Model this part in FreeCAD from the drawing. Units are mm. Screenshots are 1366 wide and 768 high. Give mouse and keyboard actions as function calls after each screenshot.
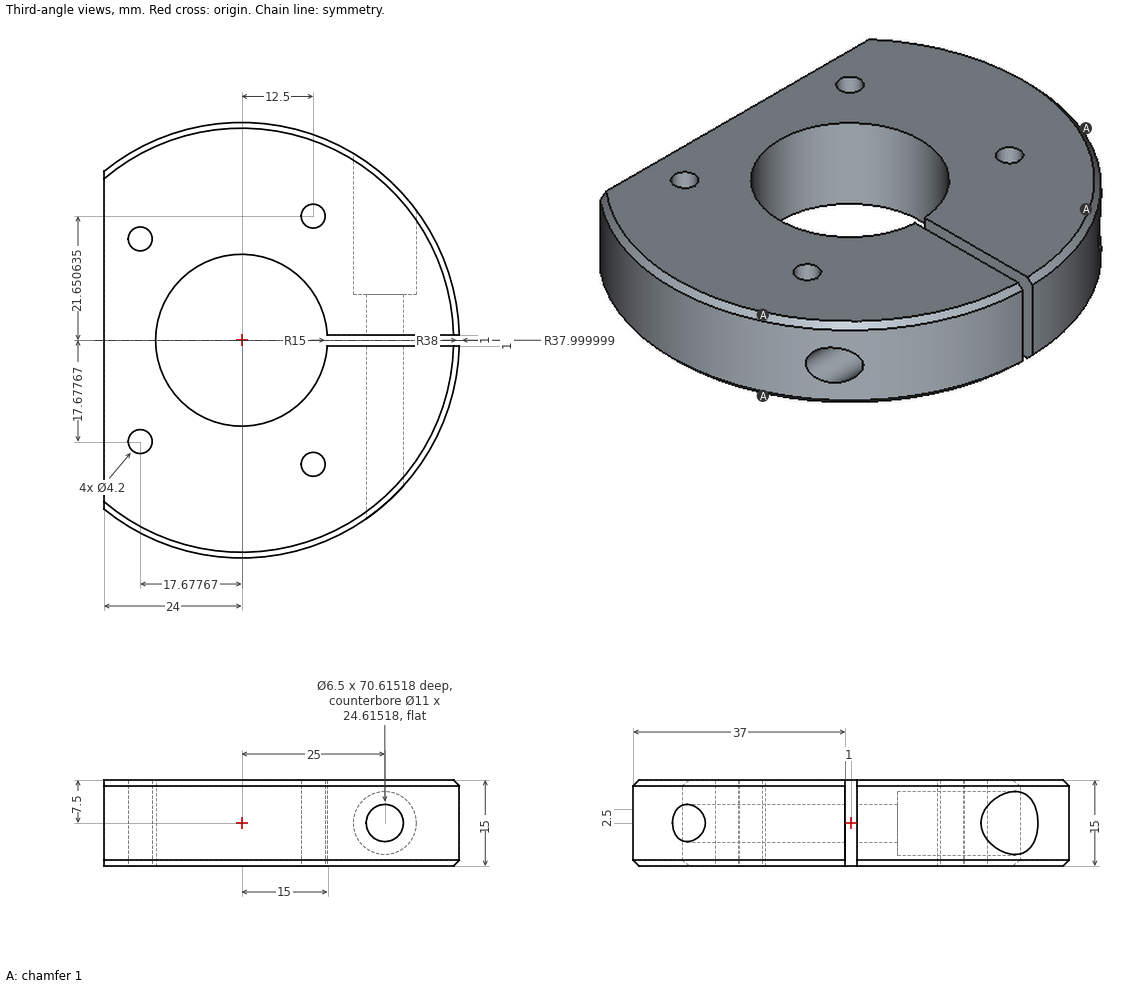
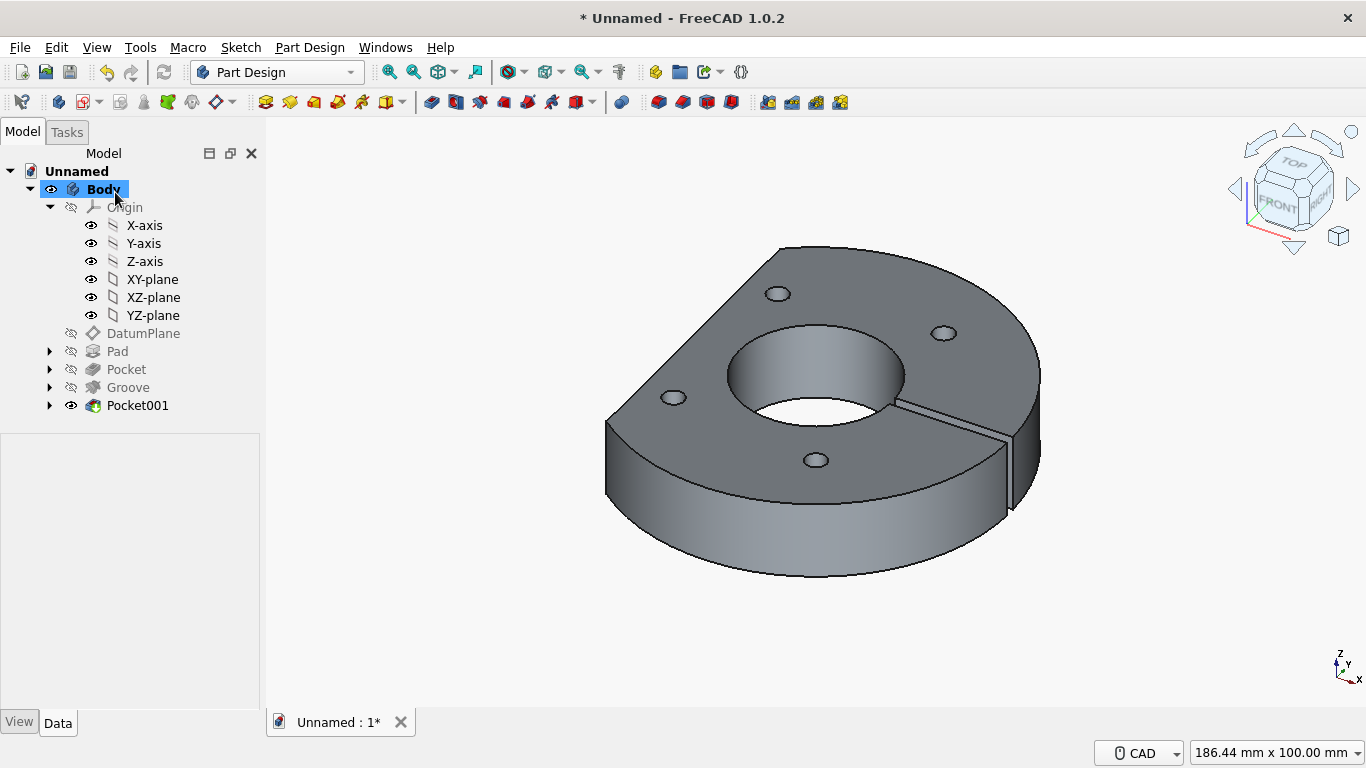
click(136, 315)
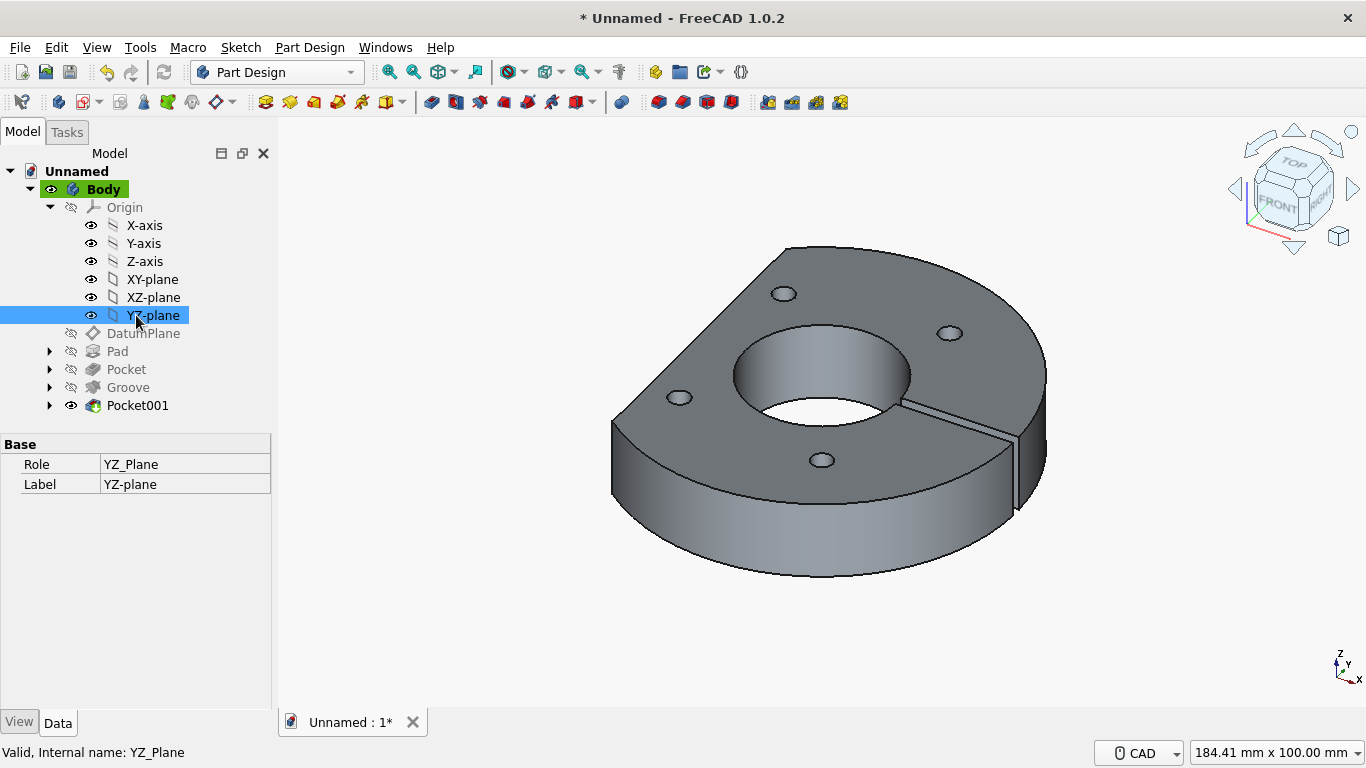
click(216, 102)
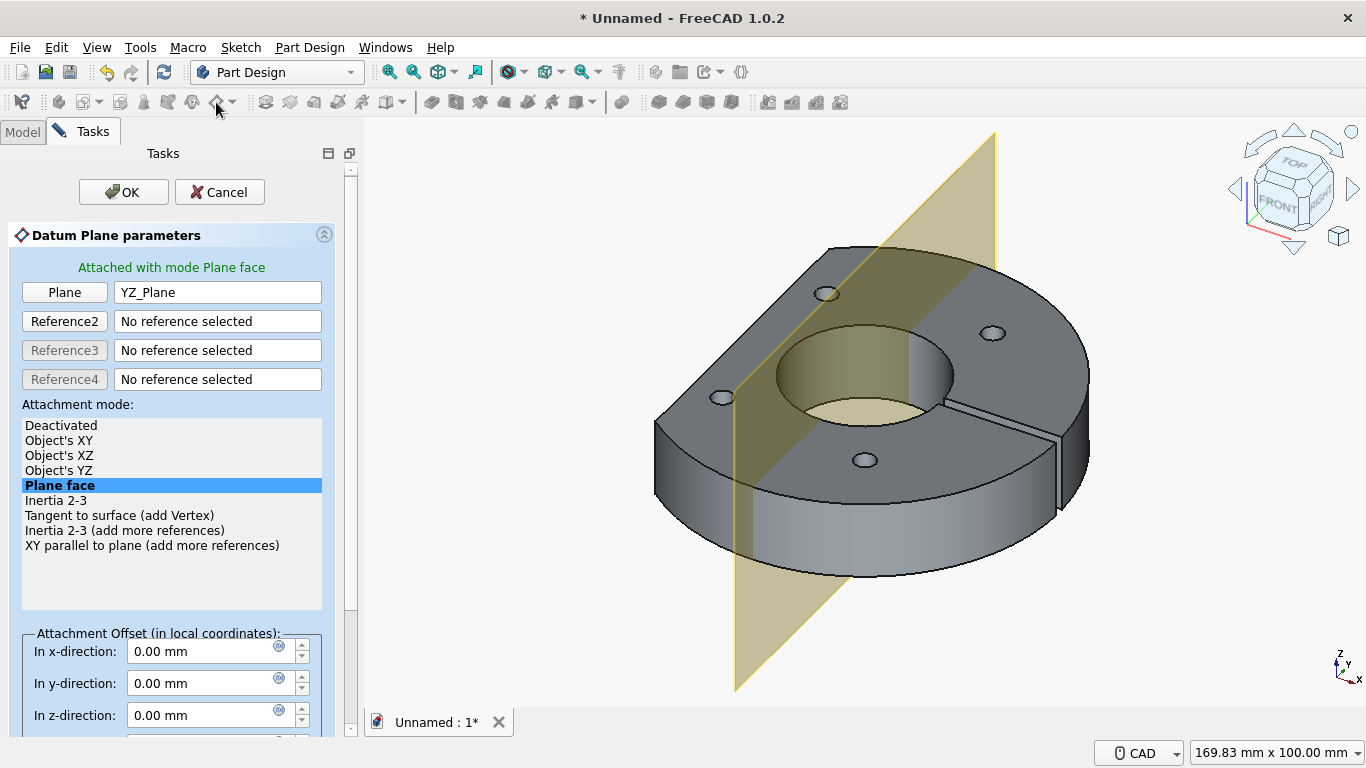
triple_click(210, 715)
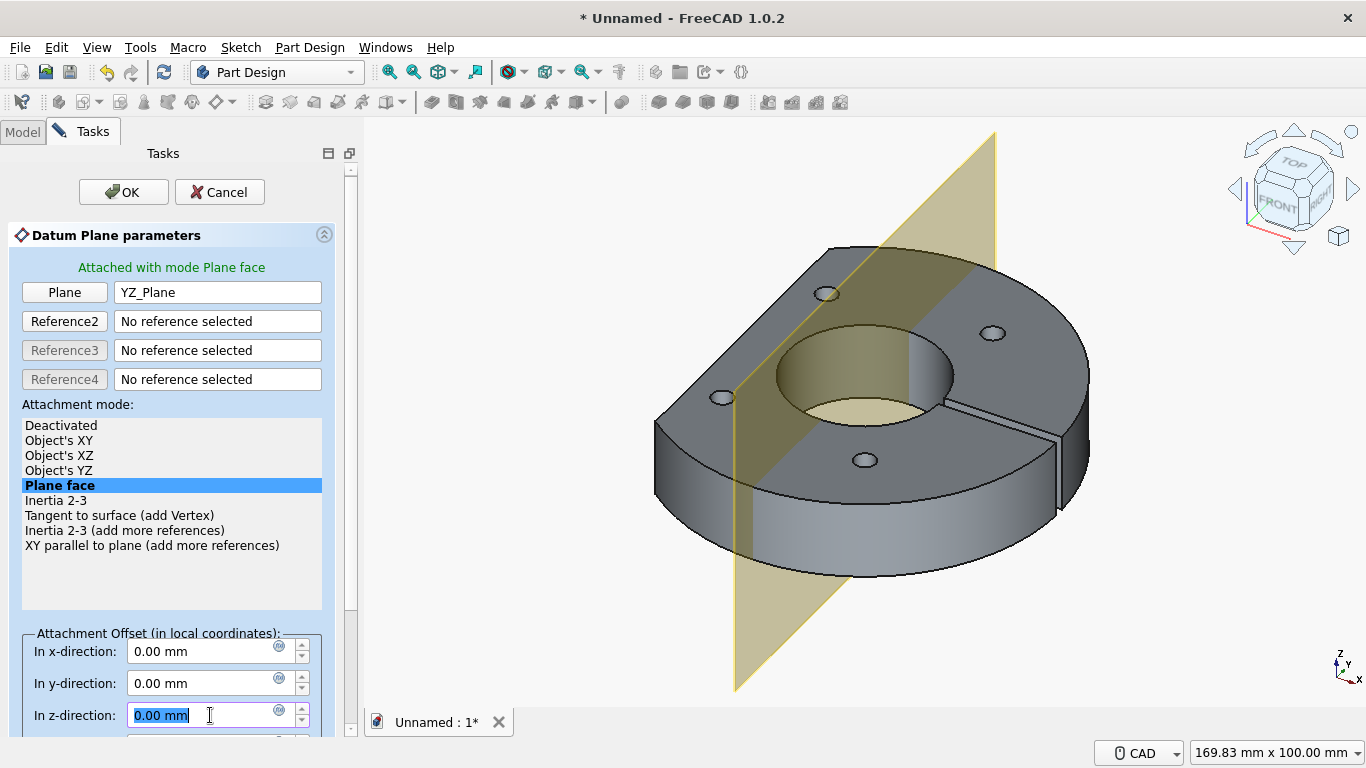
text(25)
key(Tab)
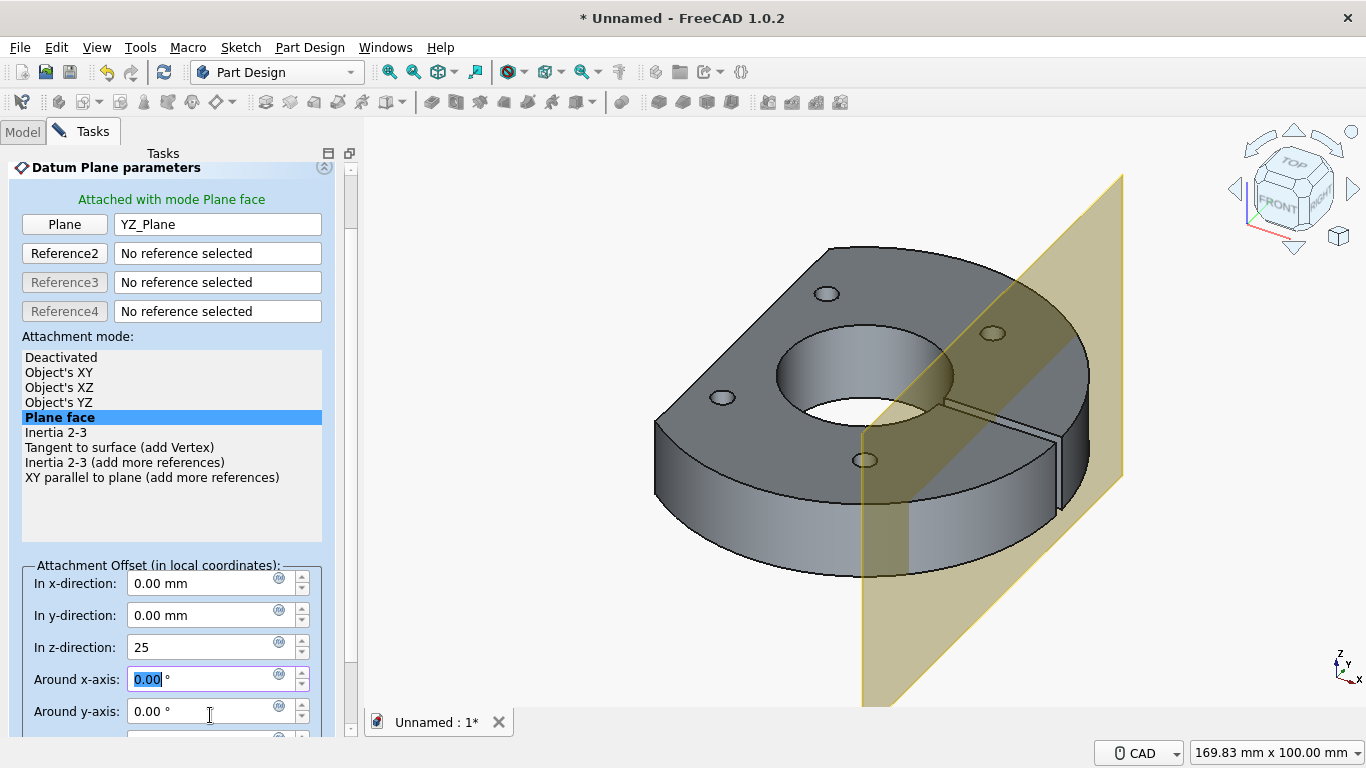
scroll(351, 450, up, 2)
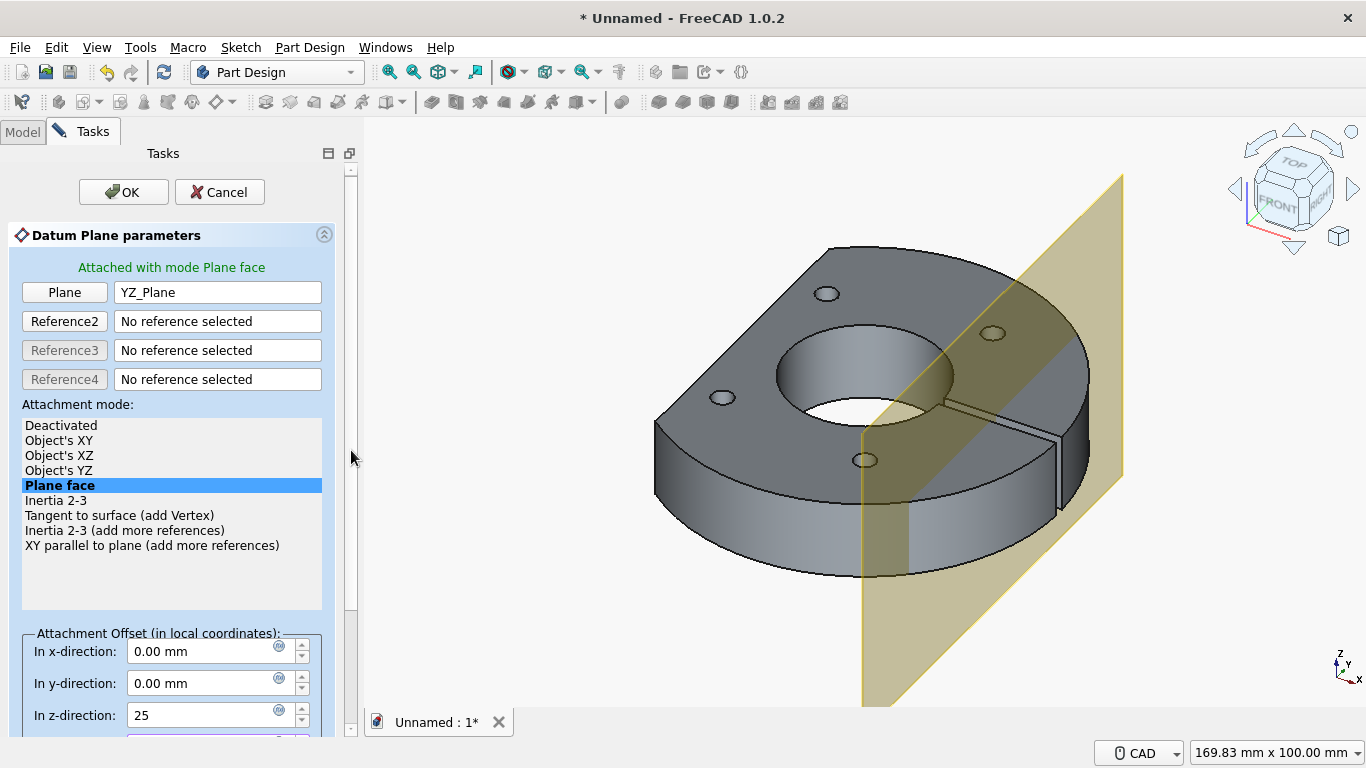
click(124, 192)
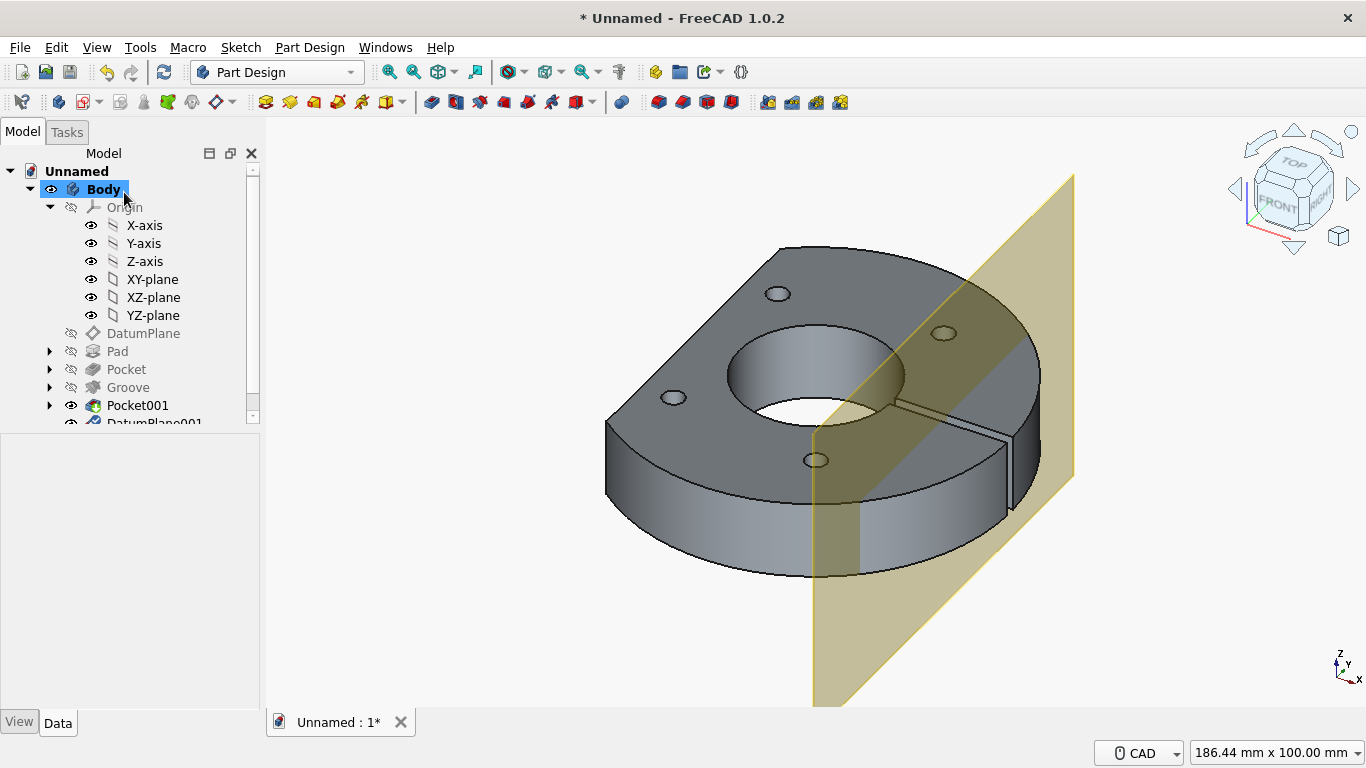
click(116, 423)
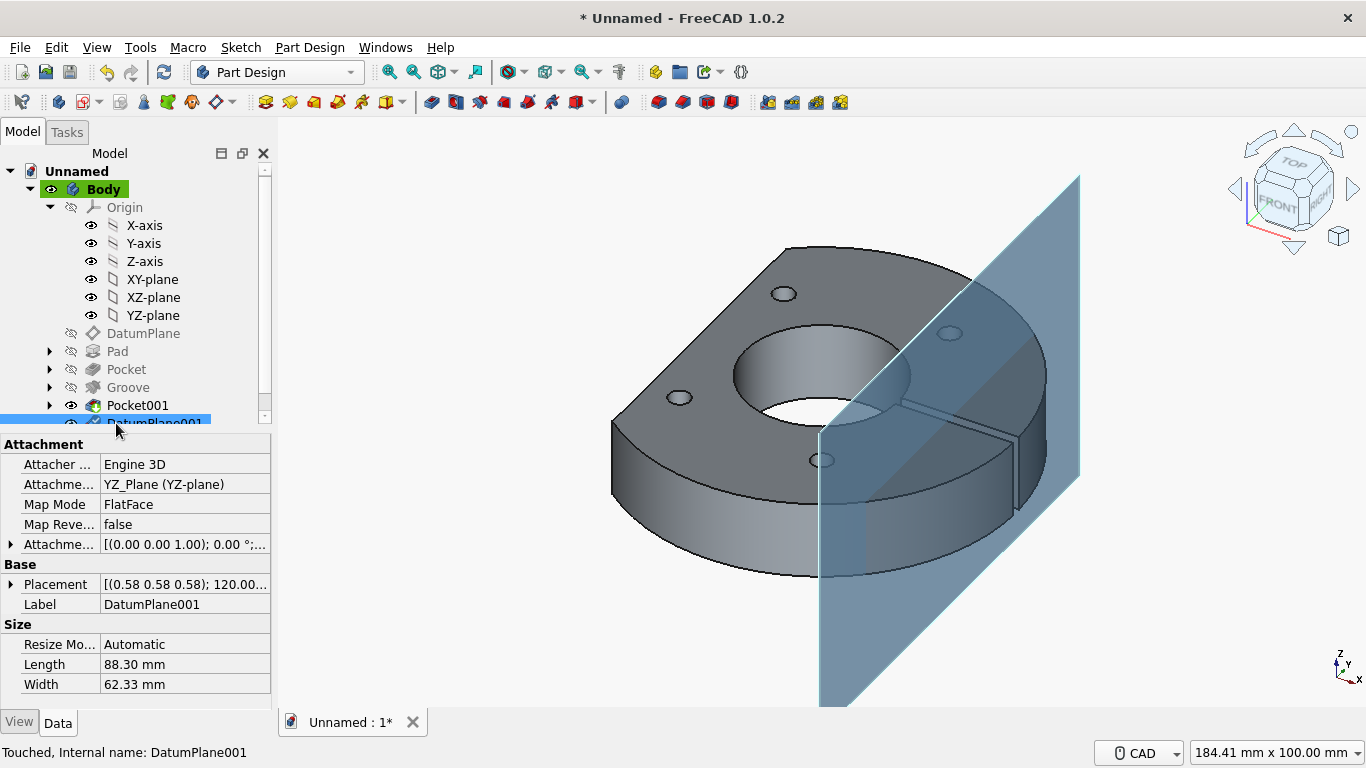
click(84, 102)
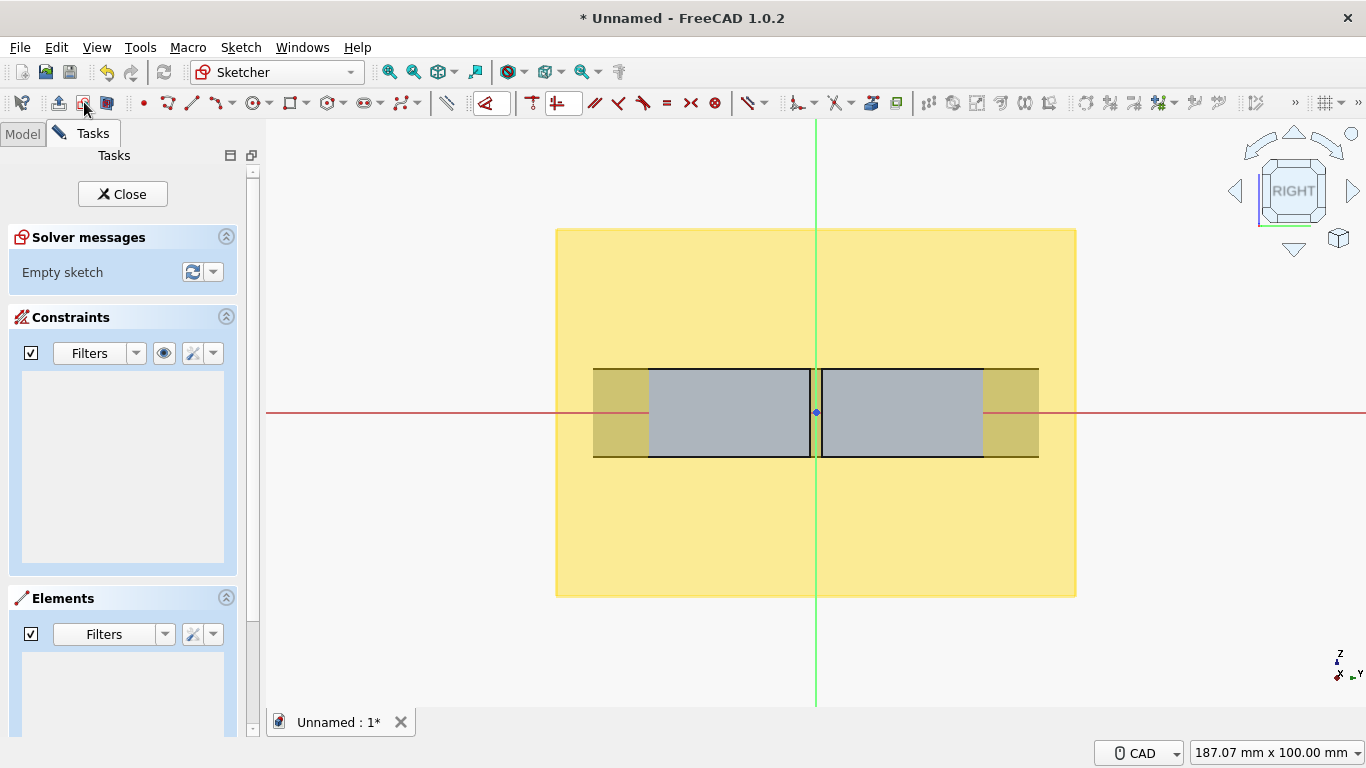
click(108, 104)